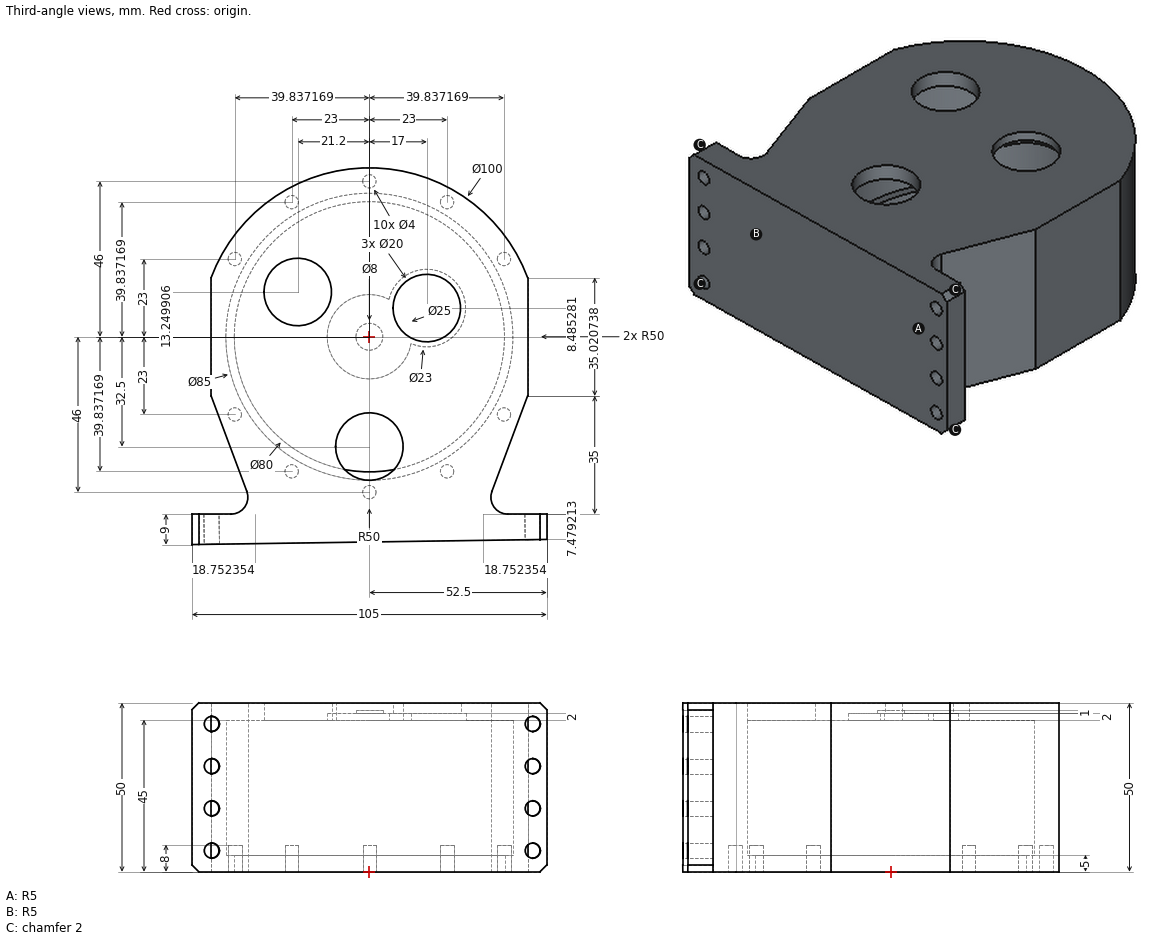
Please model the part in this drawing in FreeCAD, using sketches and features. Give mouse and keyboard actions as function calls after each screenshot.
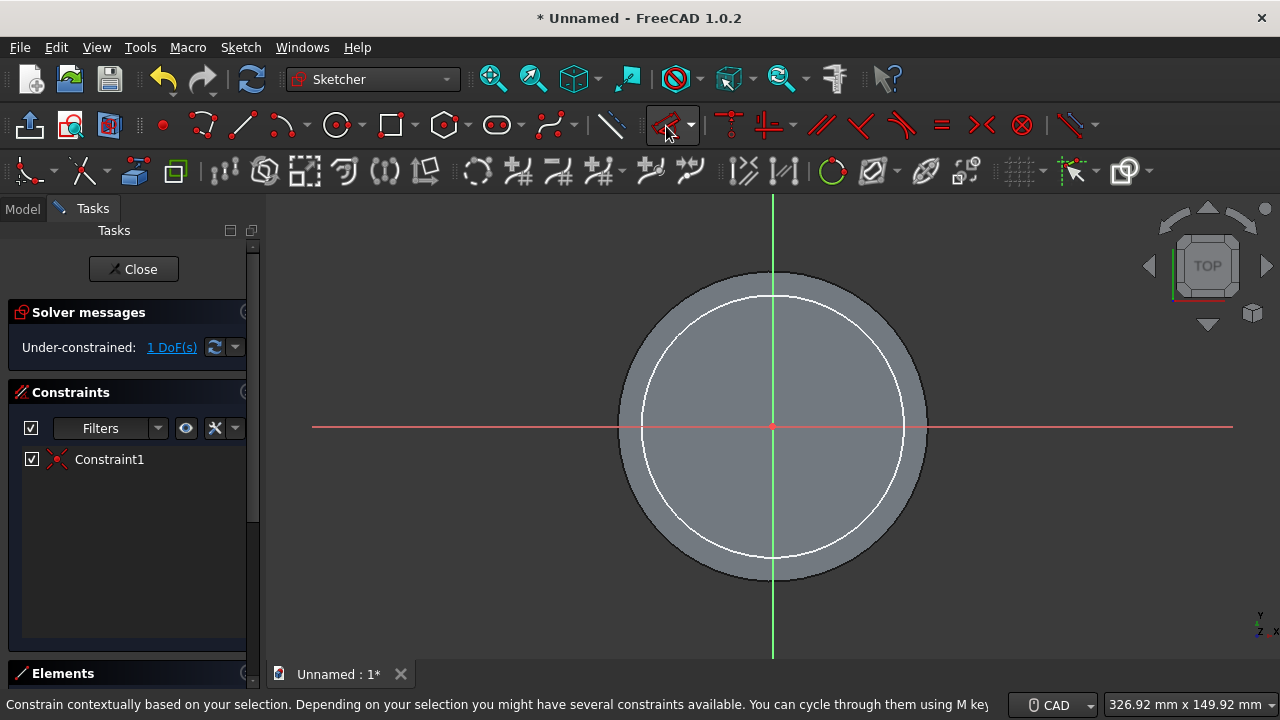
click(865, 333)
click(887, 310)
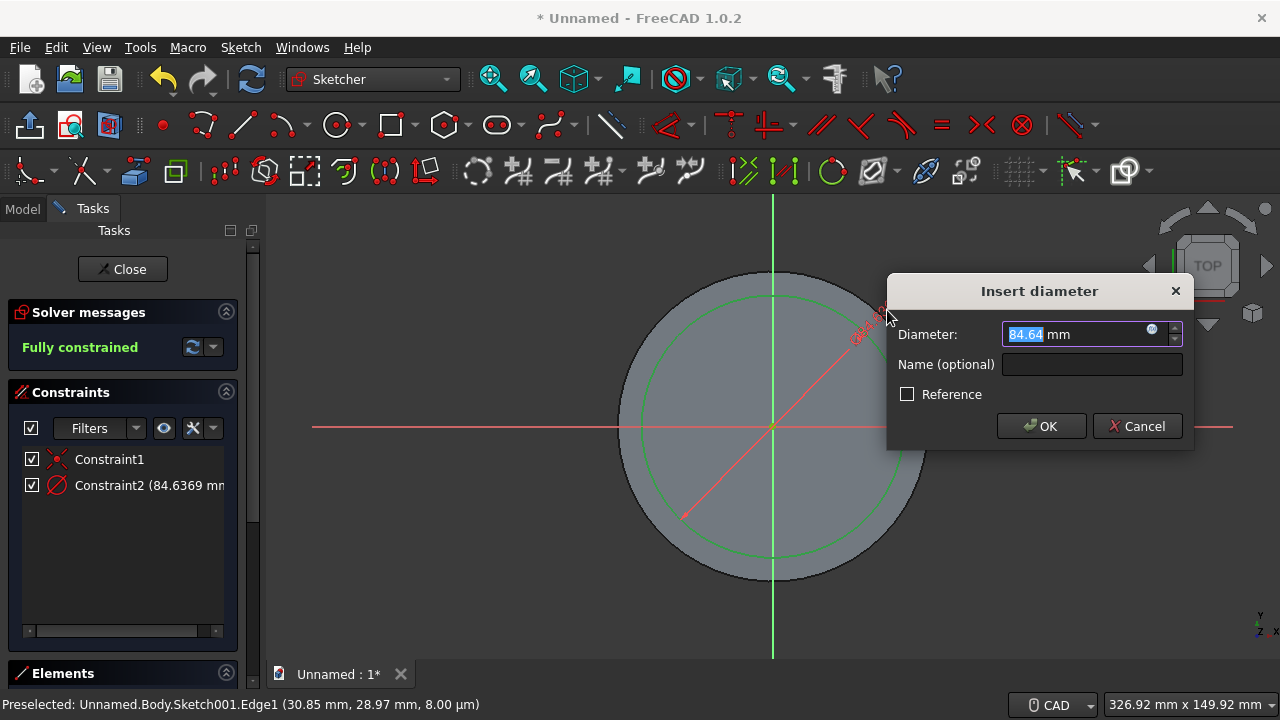
text(85)
key(Return)
key(Escape)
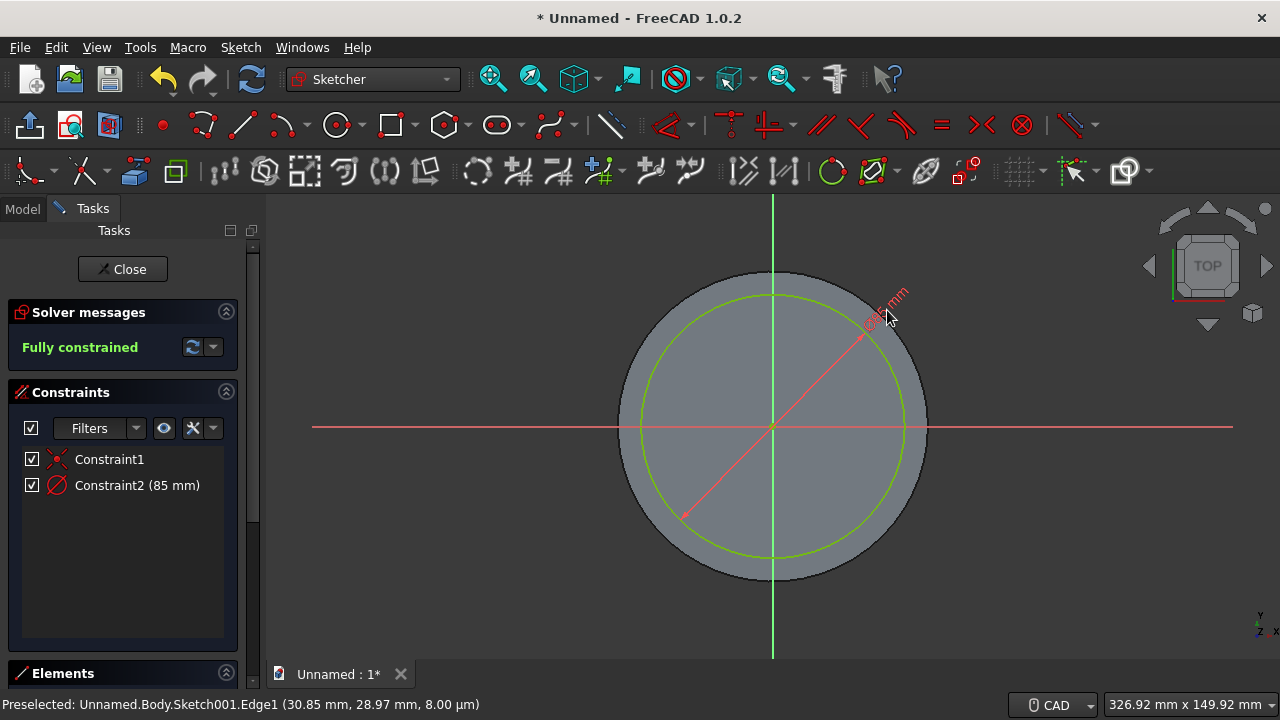
click(123, 269)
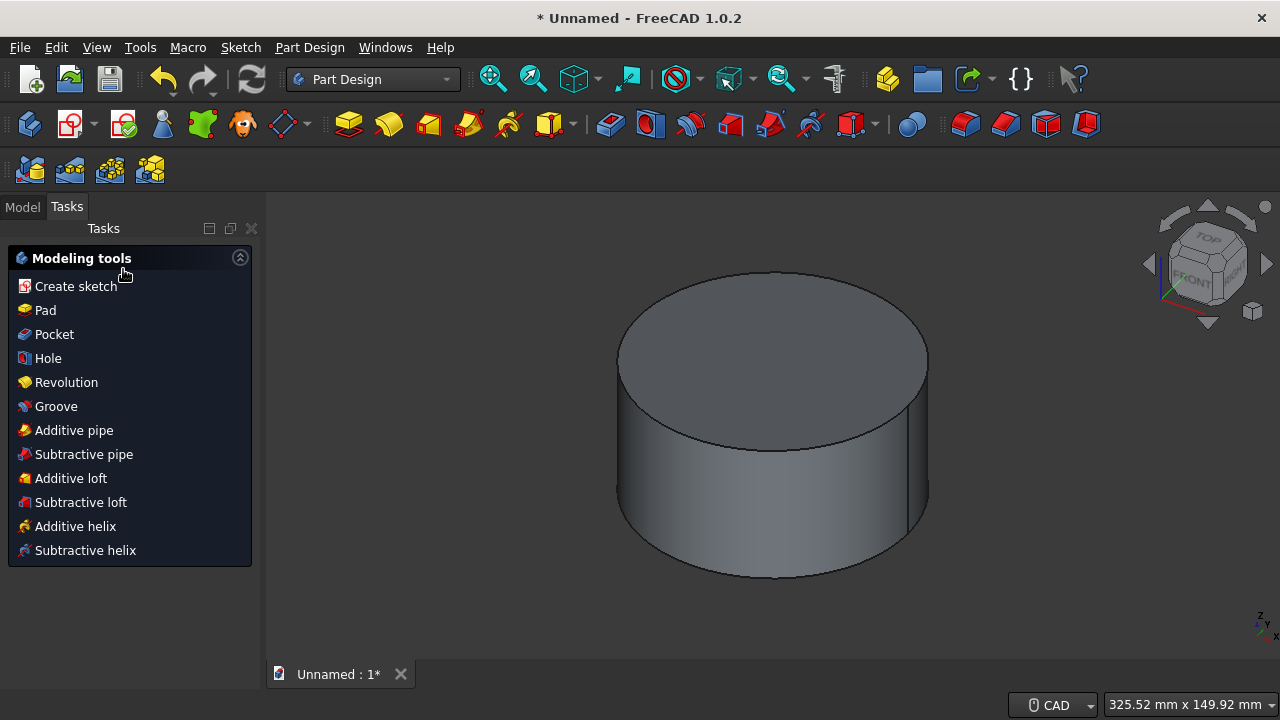
click(612, 124)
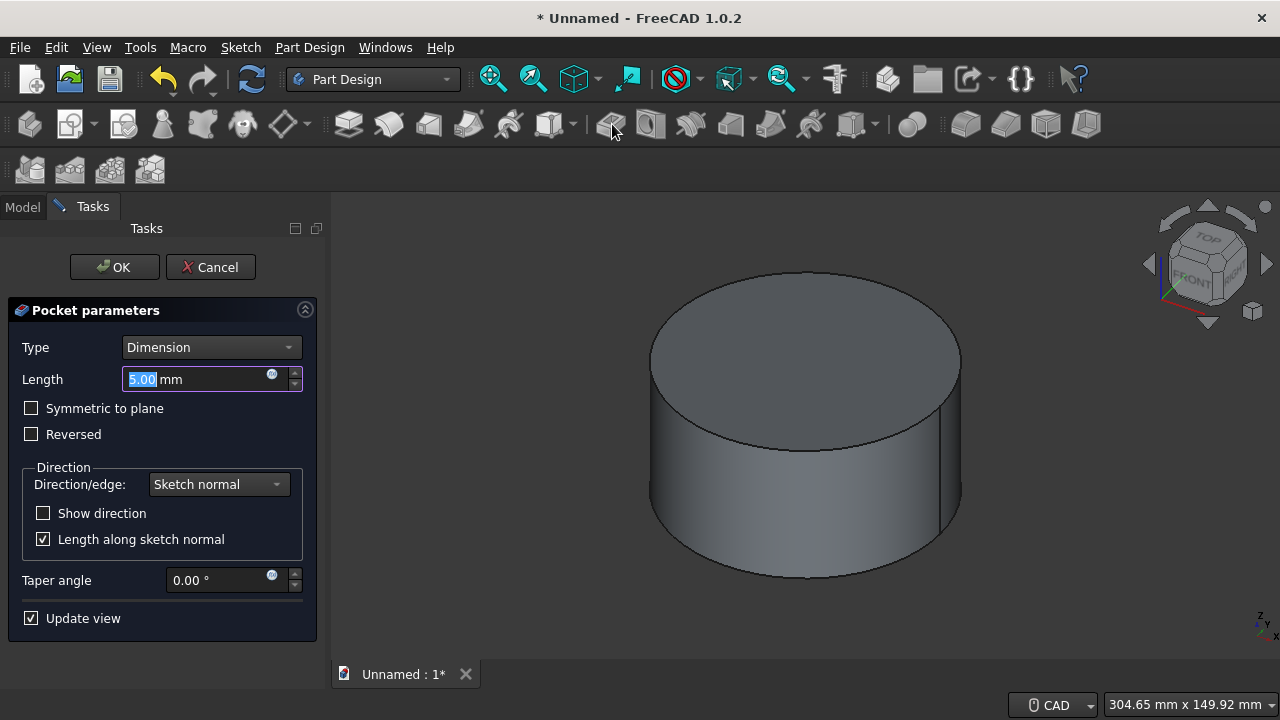
text(45)
key(Tab)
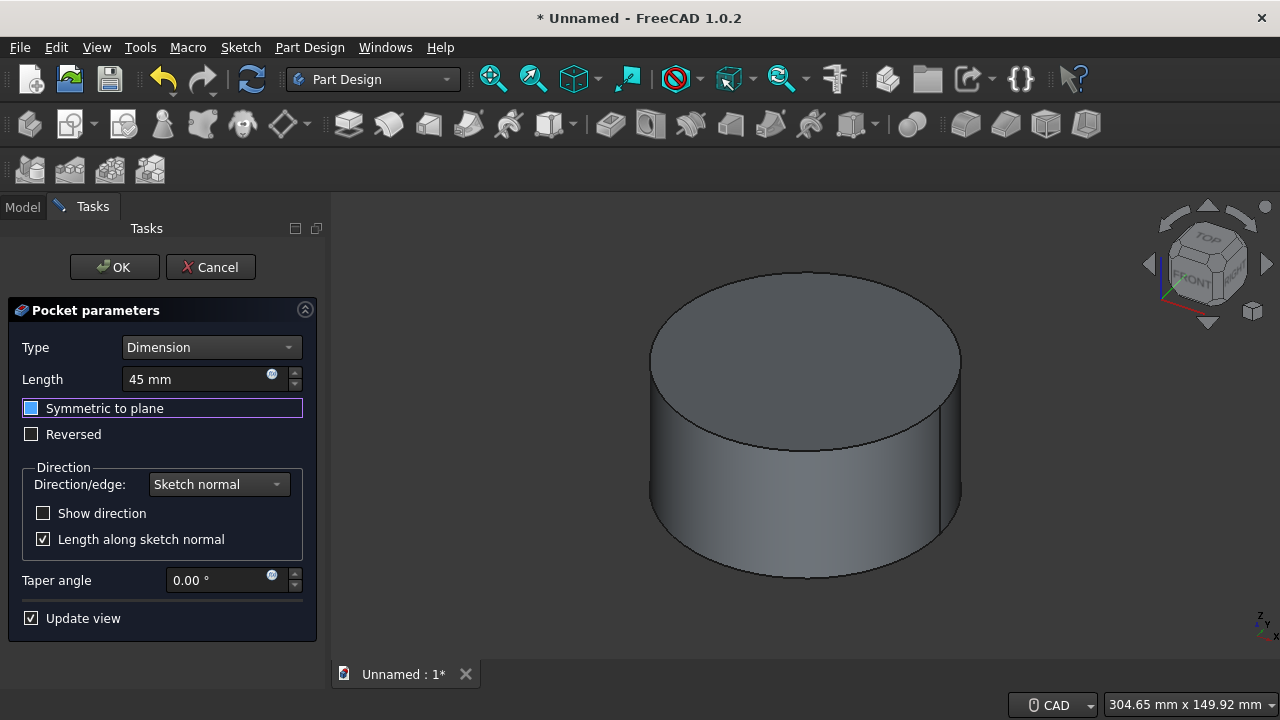
click(30, 434)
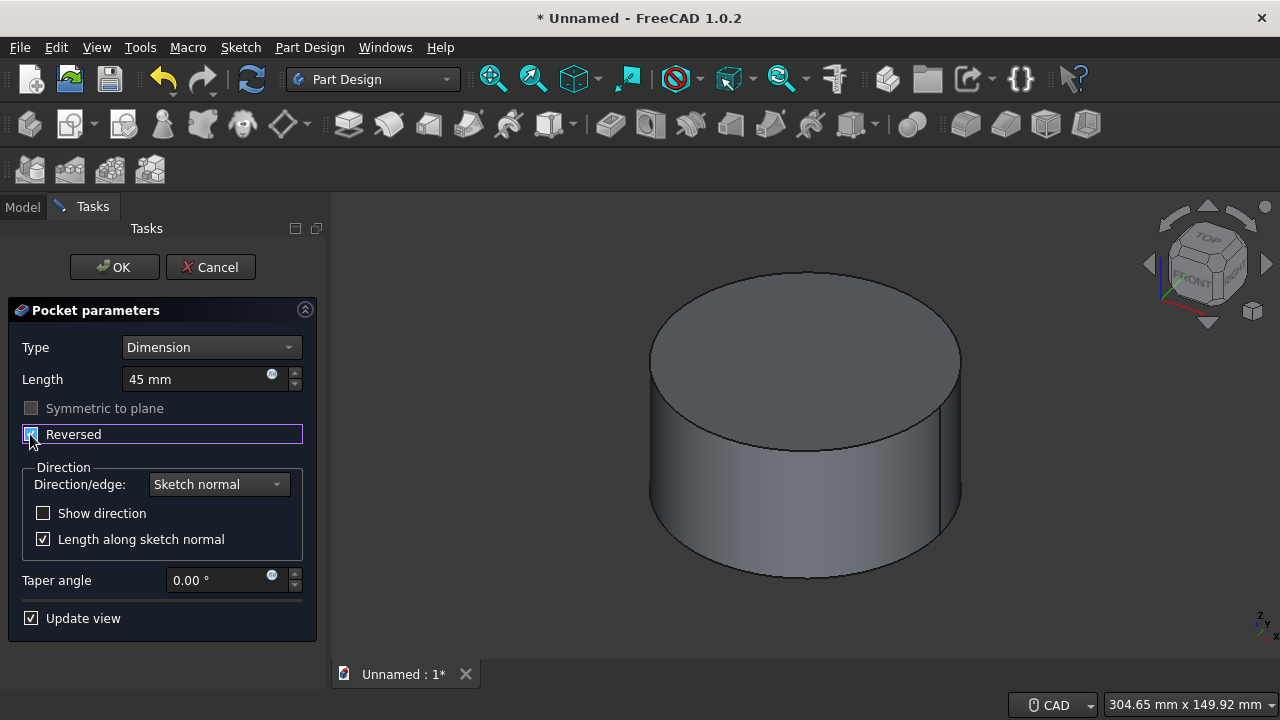
click(115, 267)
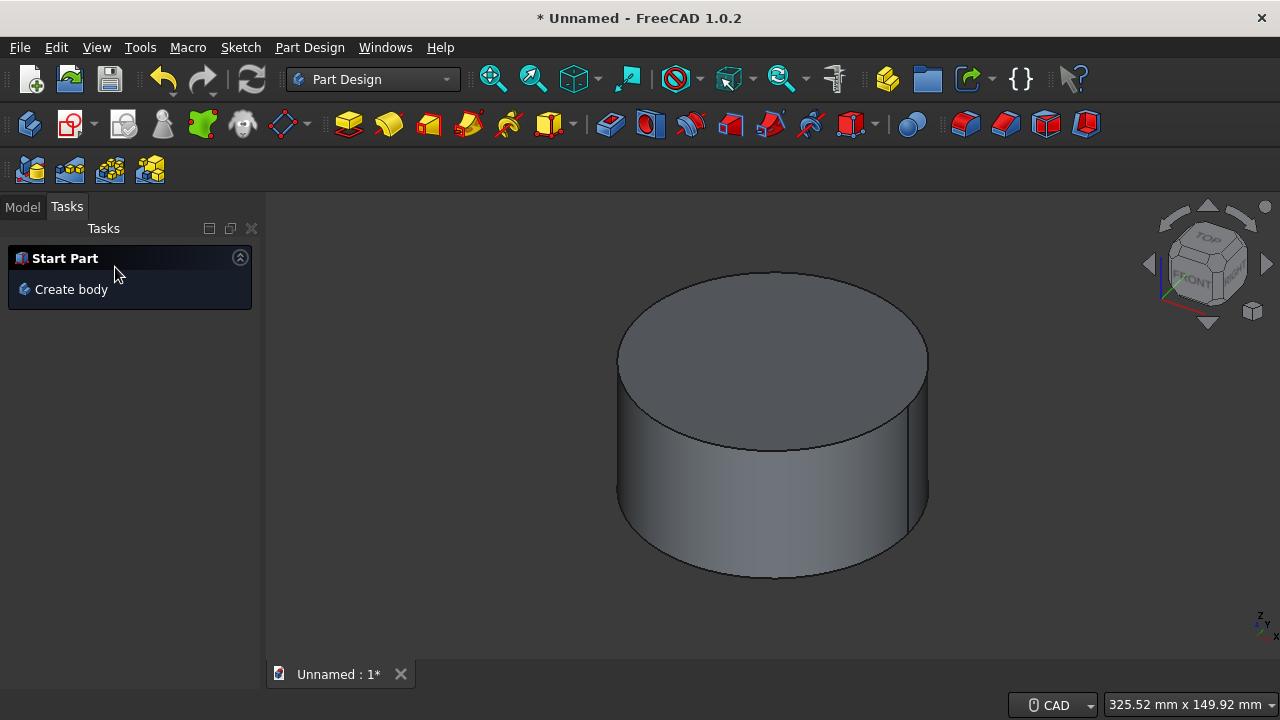
key(5)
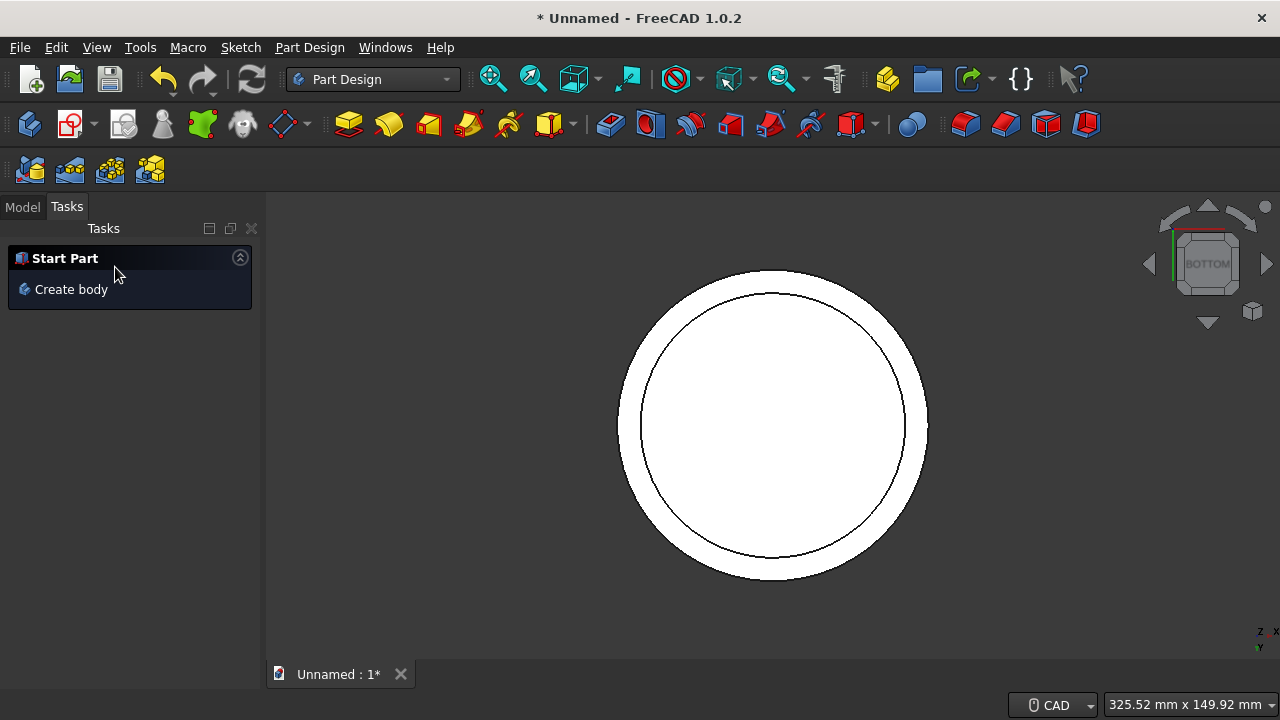
click(773, 424)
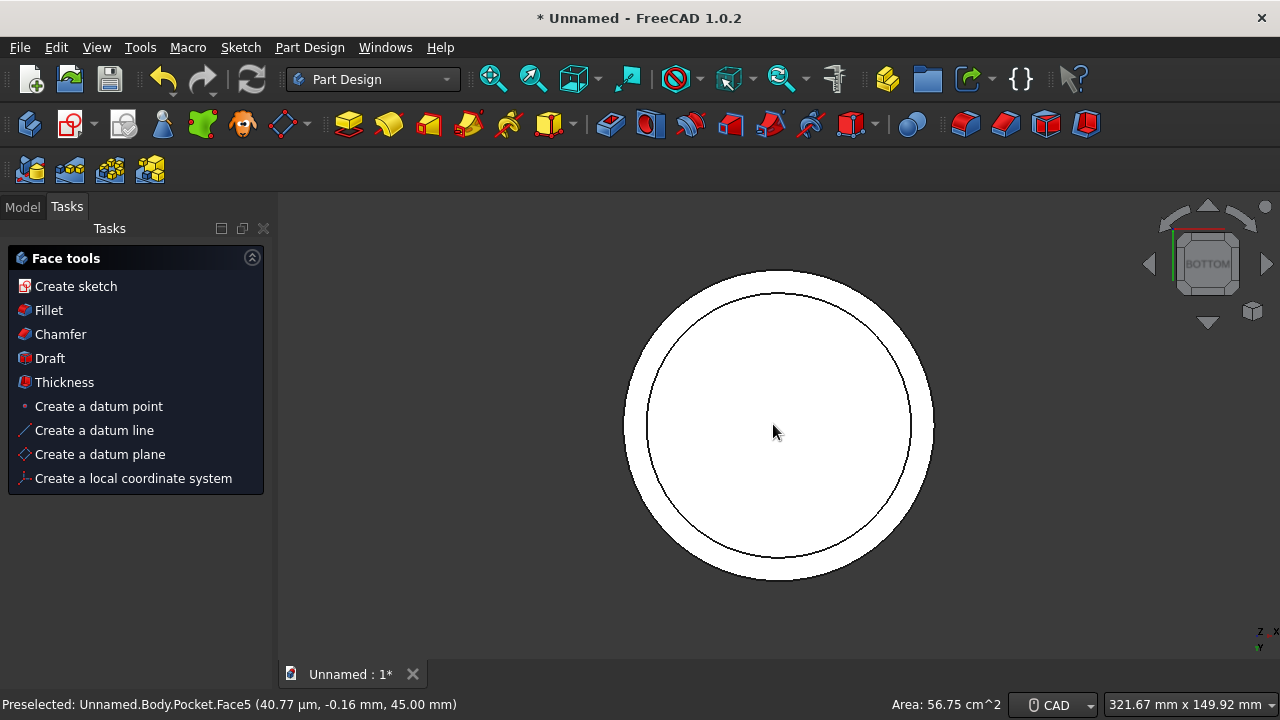
click(70, 124)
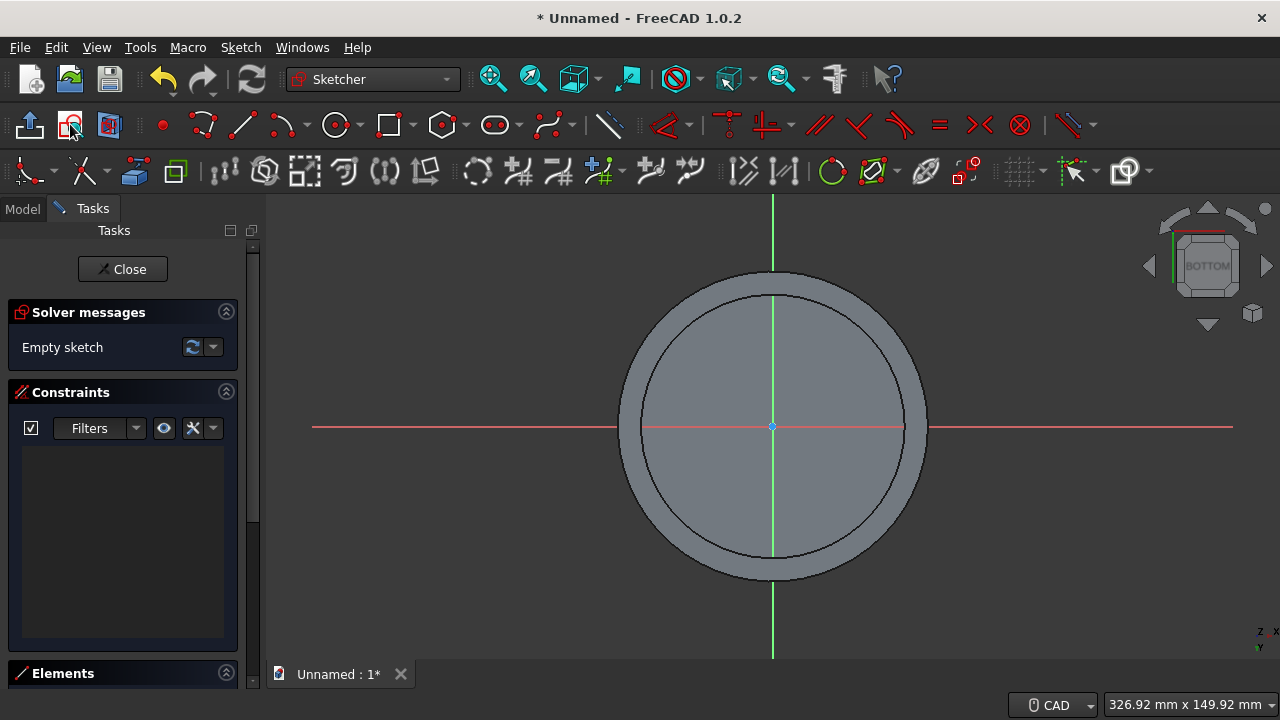
key(q)
key(s)